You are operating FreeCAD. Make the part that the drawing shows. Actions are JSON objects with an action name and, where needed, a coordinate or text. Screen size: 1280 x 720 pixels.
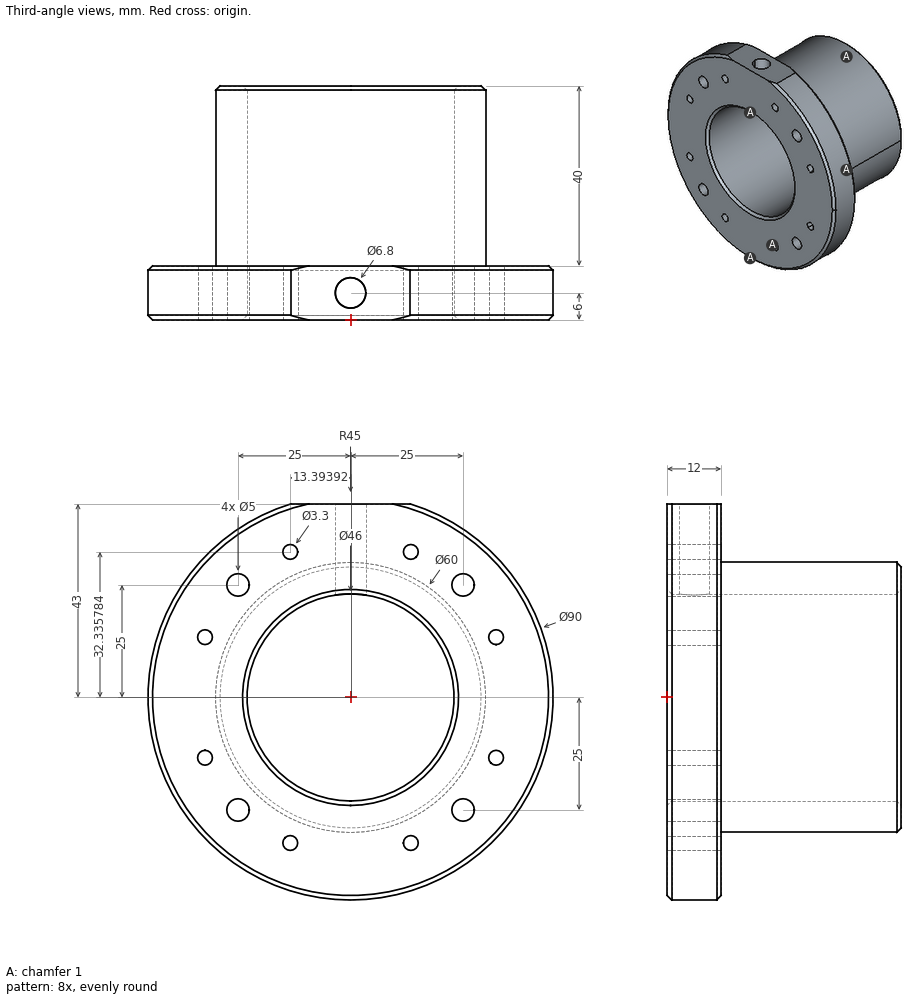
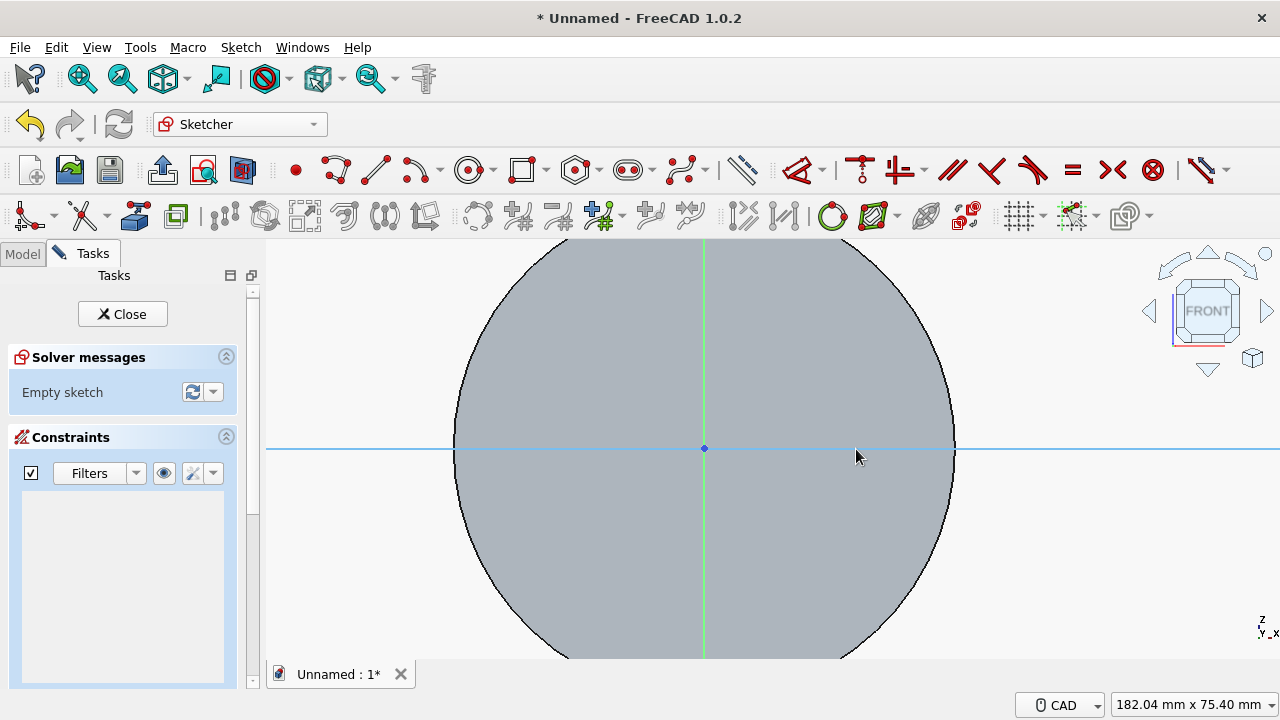
{"action": "key", "text": "g c"}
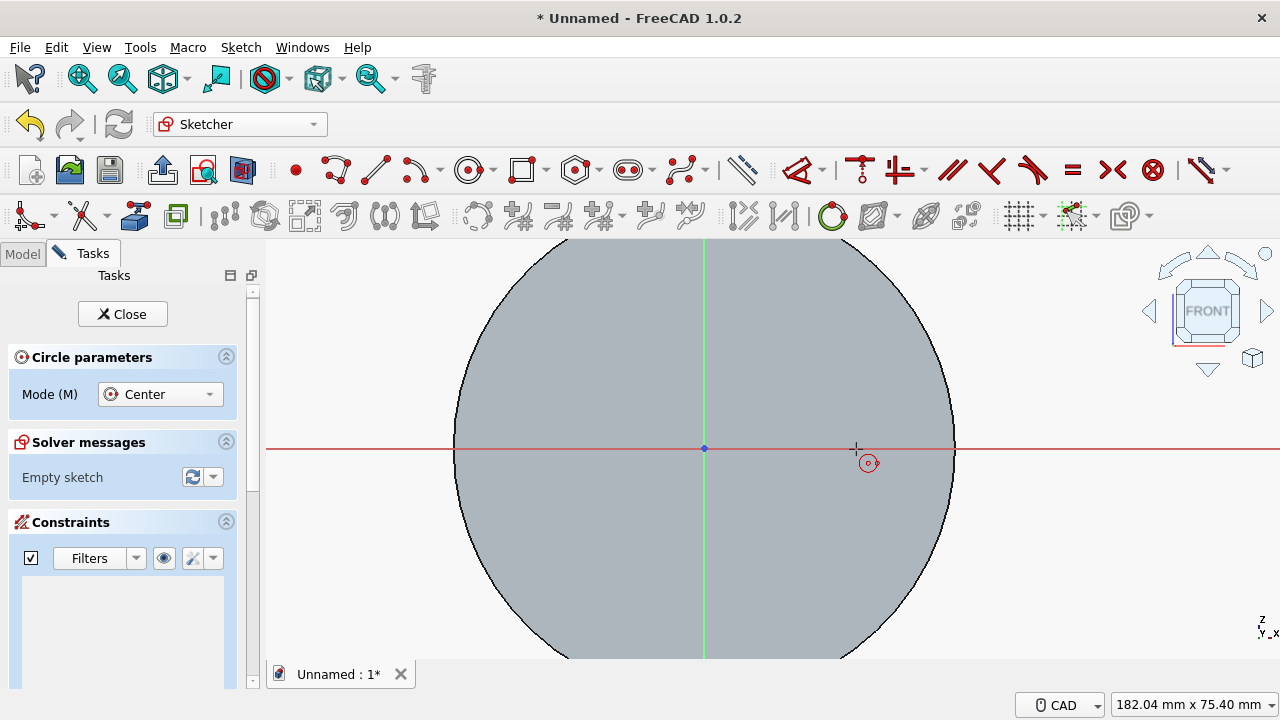
{"action": "left_click", "coordinate": [704, 449]}
{"action": "left_click", "coordinate": [795, 358]}
{"action": "key", "text": "Escape"}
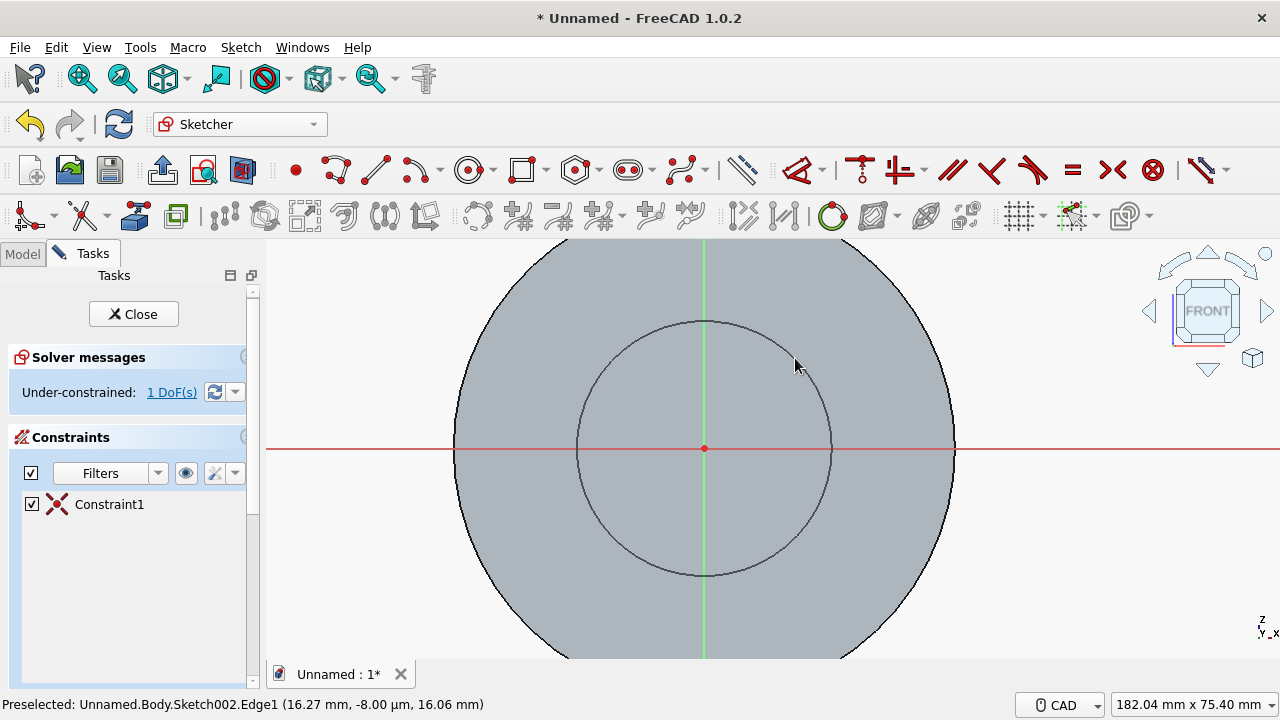
{"action": "key", "text": "d"}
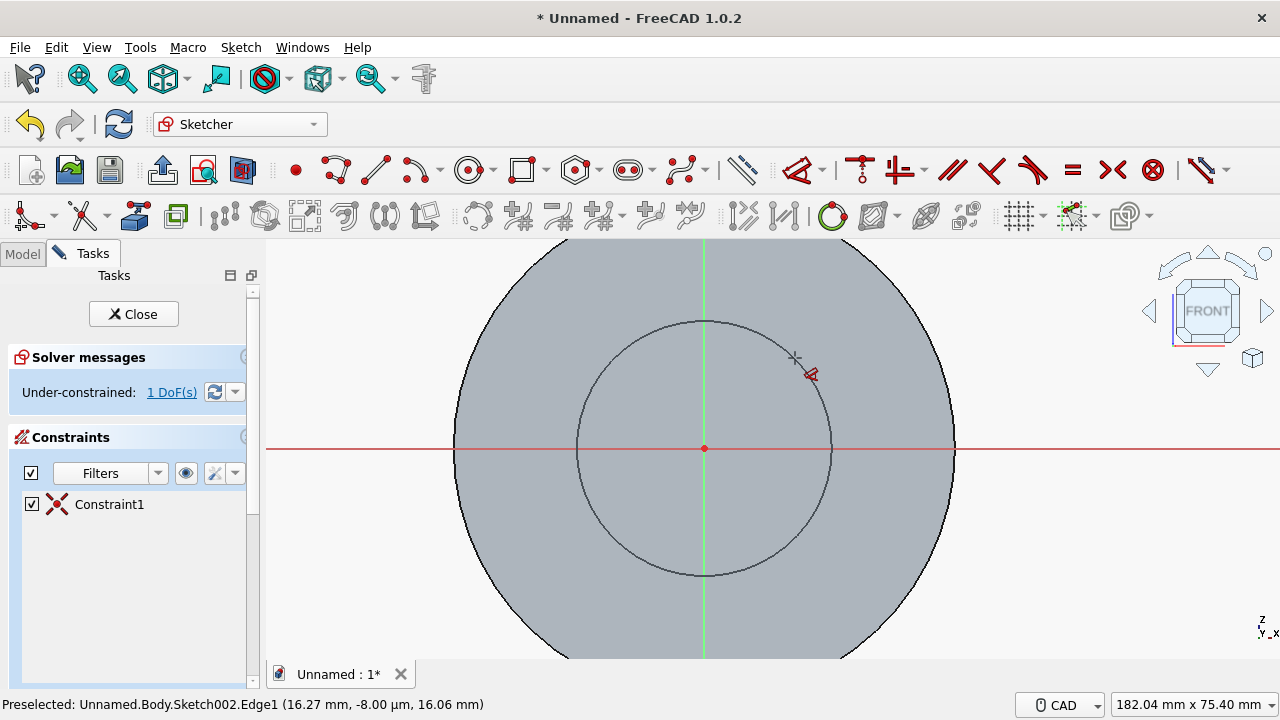
{"action": "left_click", "coordinate": [794, 358]}
{"action": "left_click", "coordinate": [817, 335]}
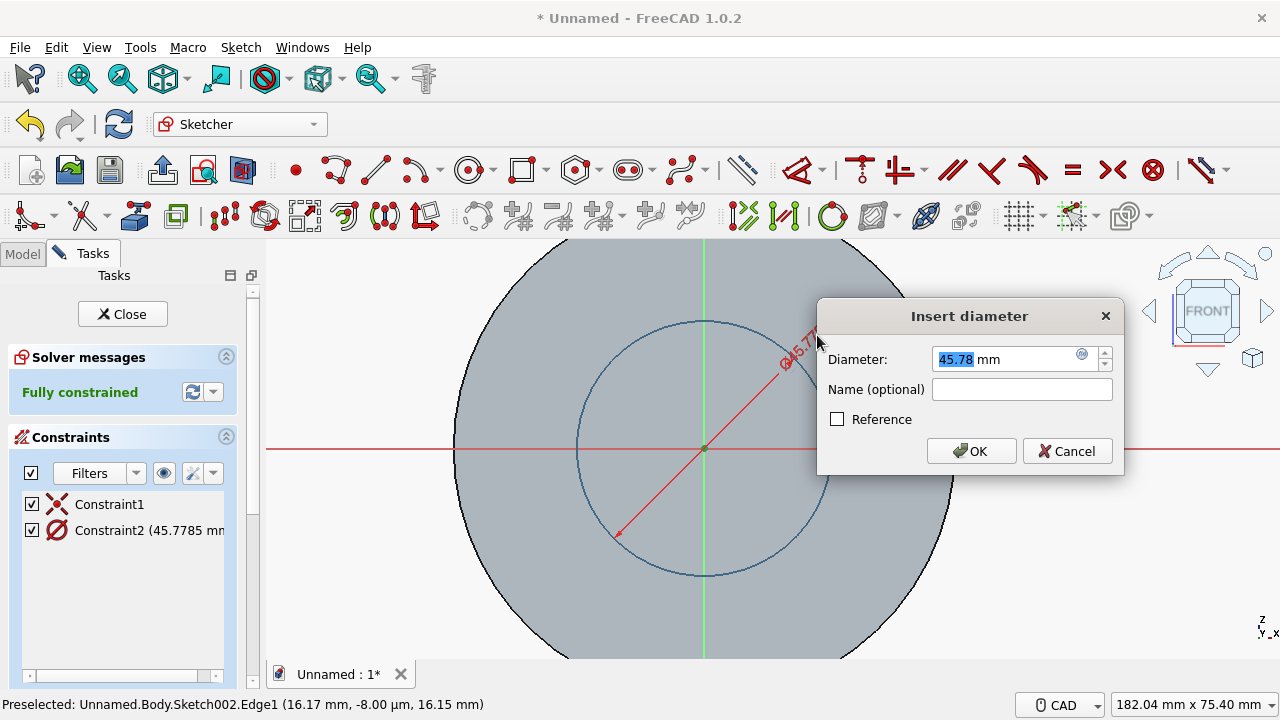
{"action": "type", "text": "46"}
{"action": "key", "text": "Return"}
{"action": "key", "text": "Escape"}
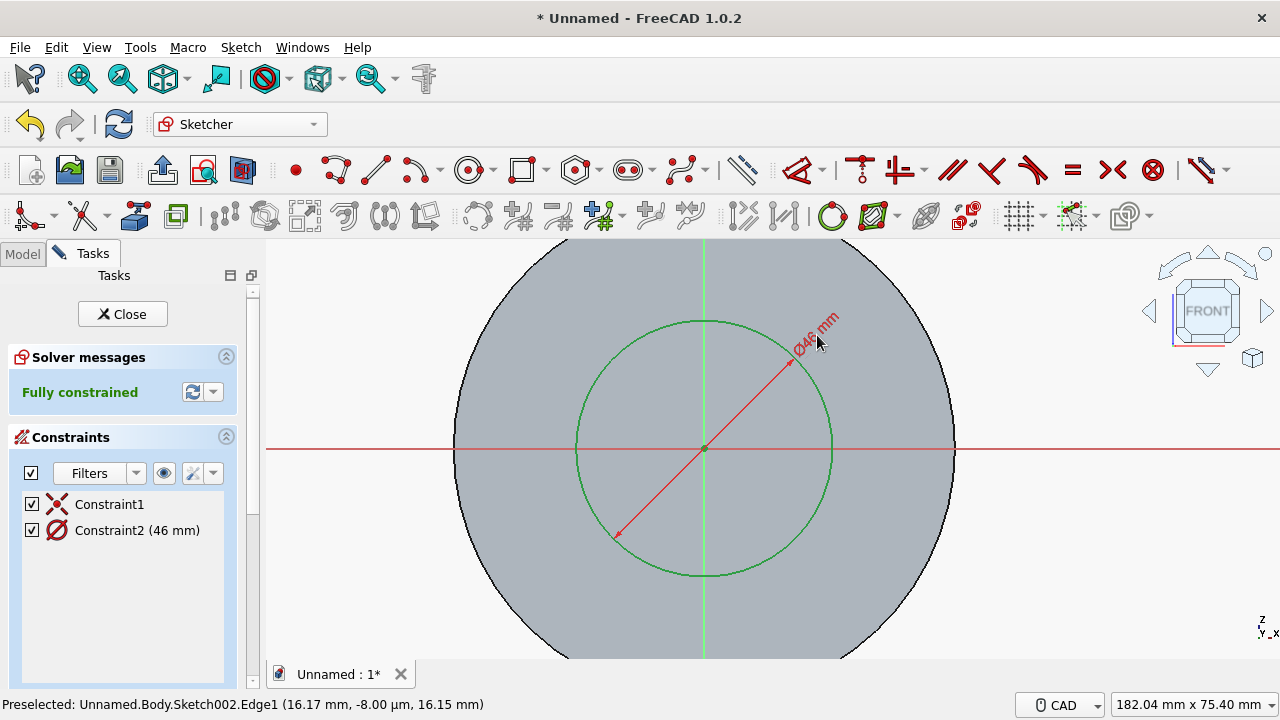
{"action": "left_click", "coordinate": [123, 314]}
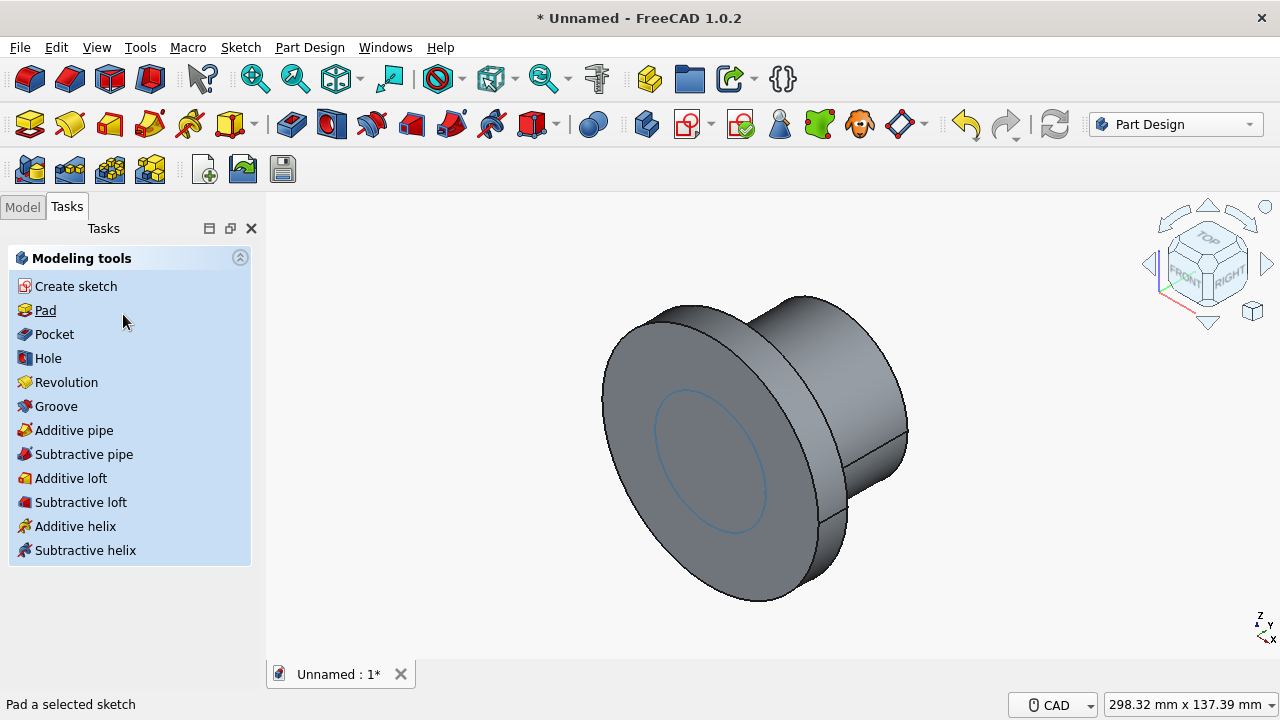
{"action": "left_click", "coordinate": [292, 124]}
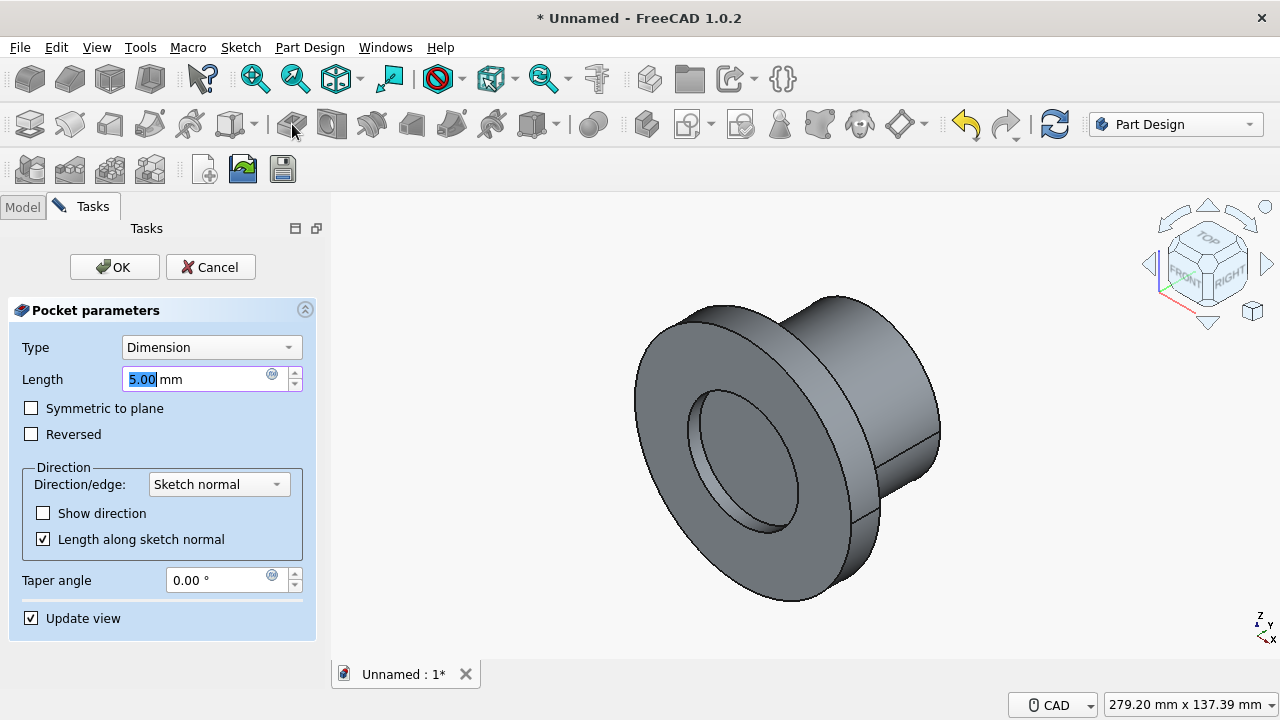
{"action": "left_click", "coordinate": [212, 348]}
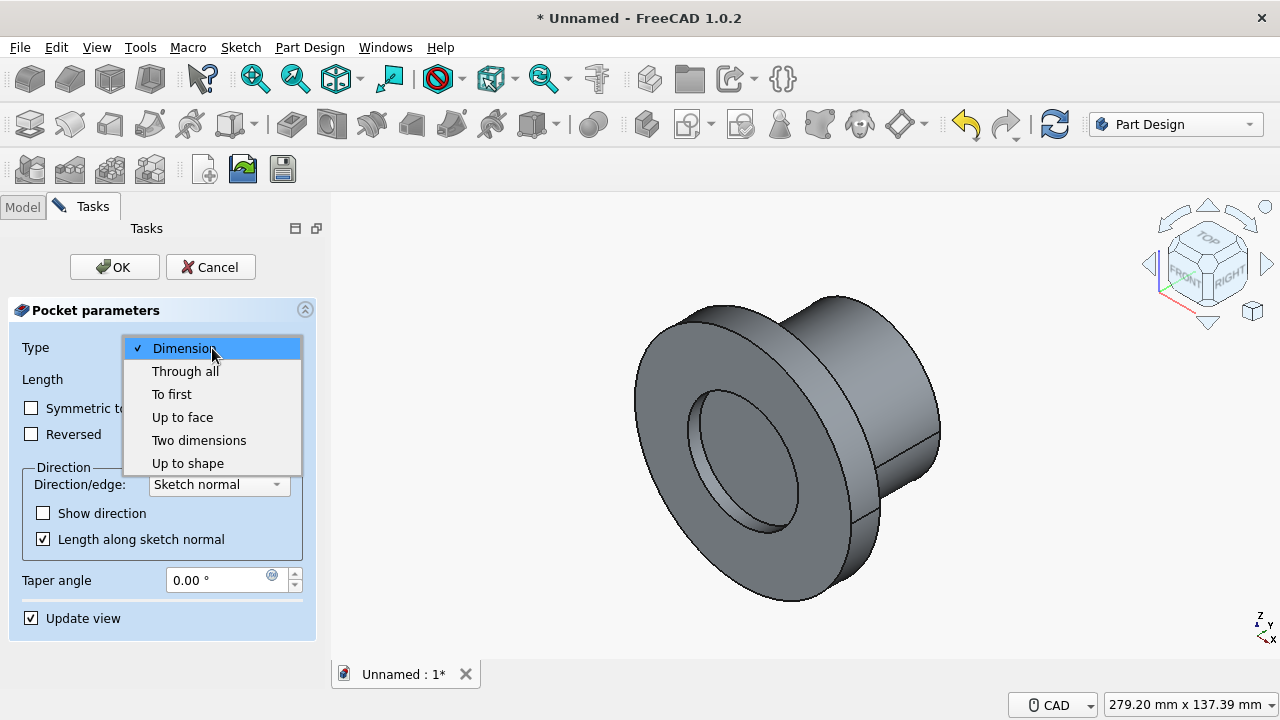
{"action": "left_click", "coordinate": [212, 372]}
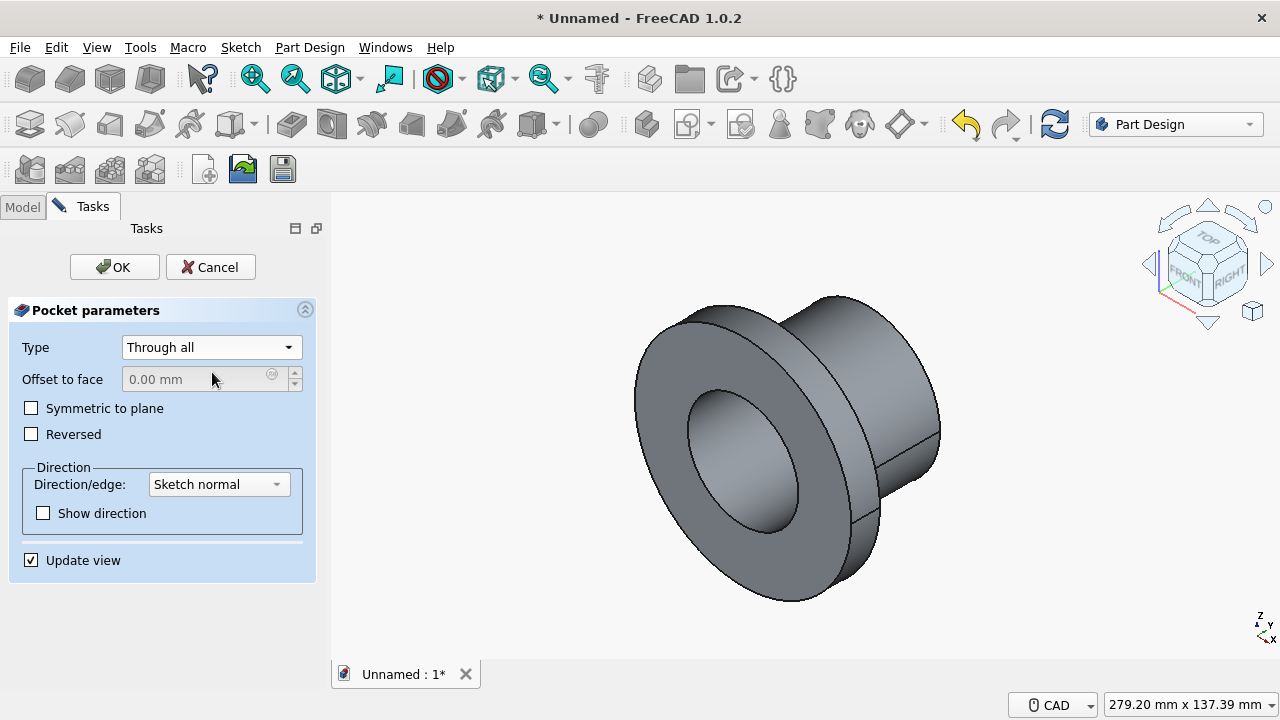
{"action": "left_click", "coordinate": [115, 267]}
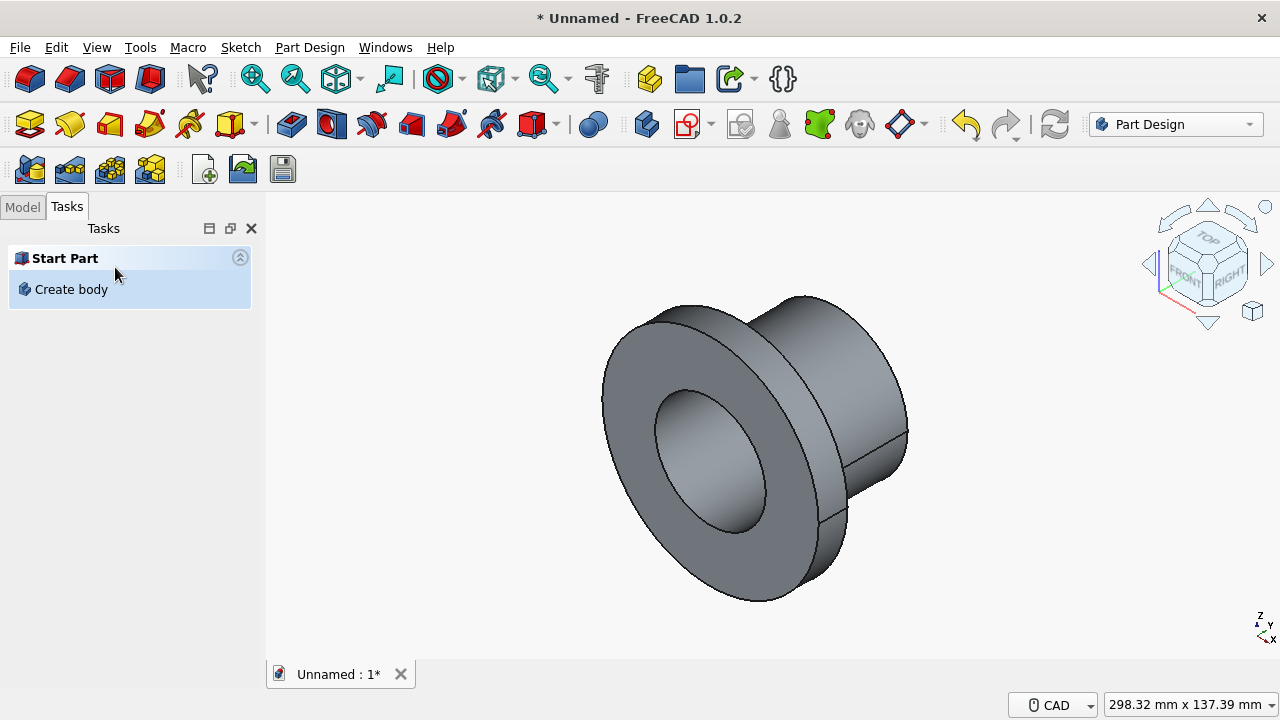
{"action": "left_click", "coordinate": [655, 429]}